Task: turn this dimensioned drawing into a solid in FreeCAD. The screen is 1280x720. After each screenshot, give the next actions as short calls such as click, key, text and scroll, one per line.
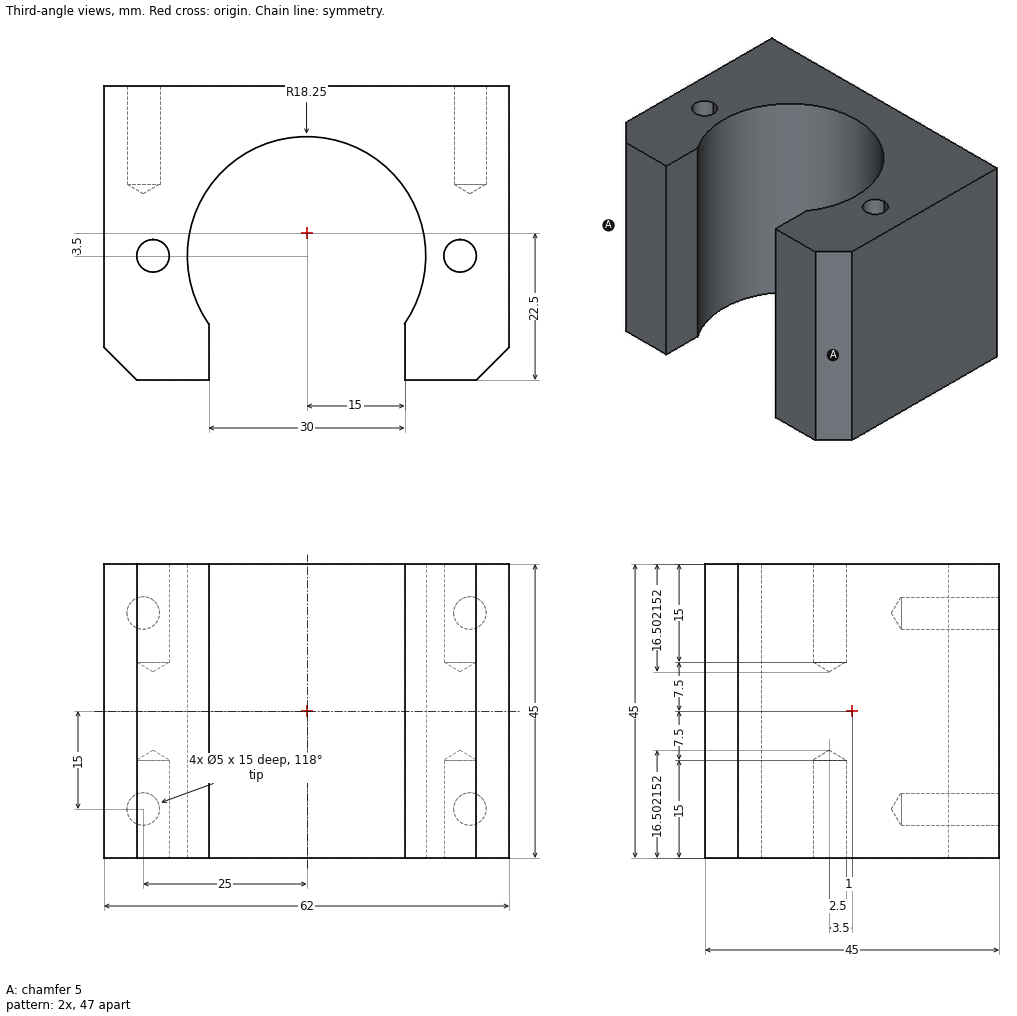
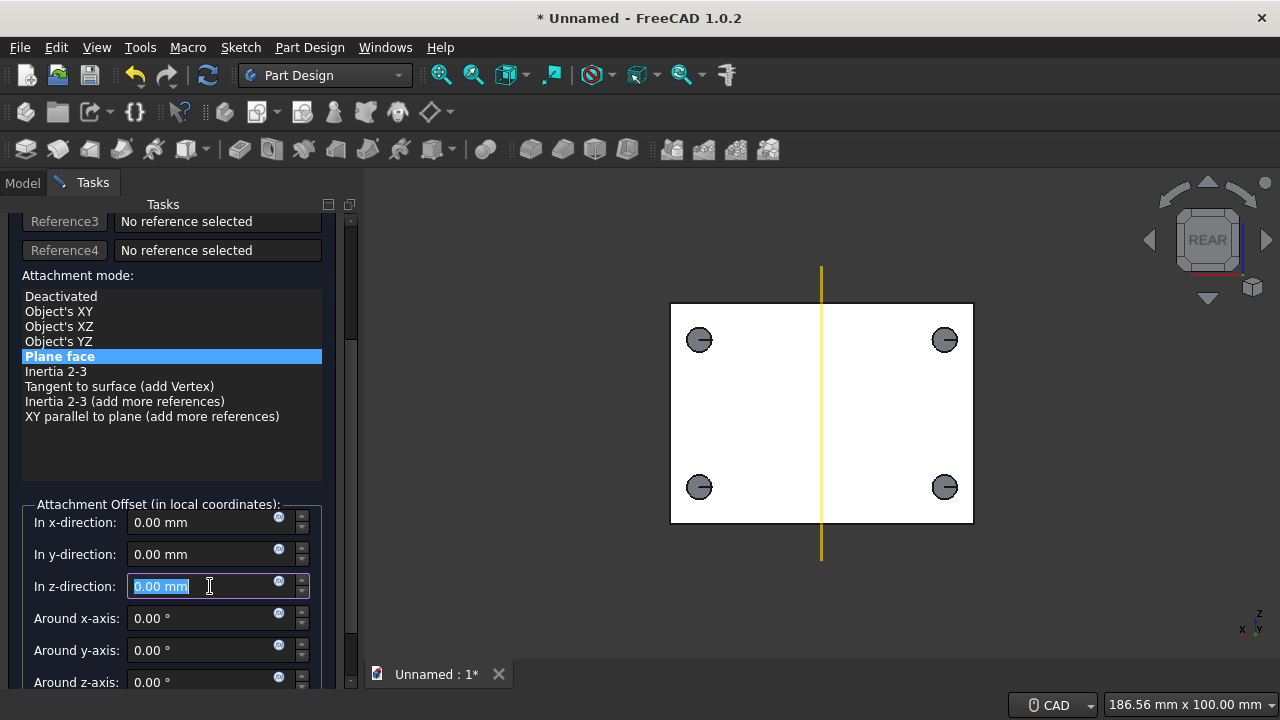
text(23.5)
key(Tab)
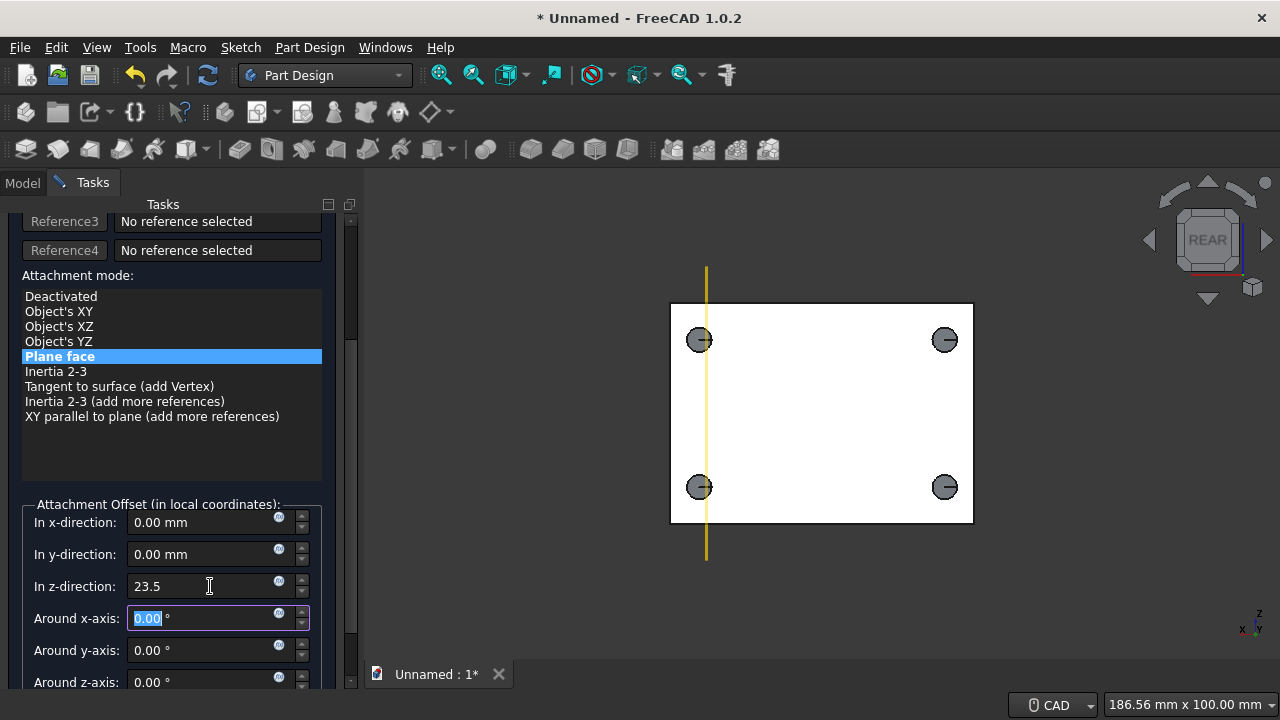
scroll(351, 451, up, 4)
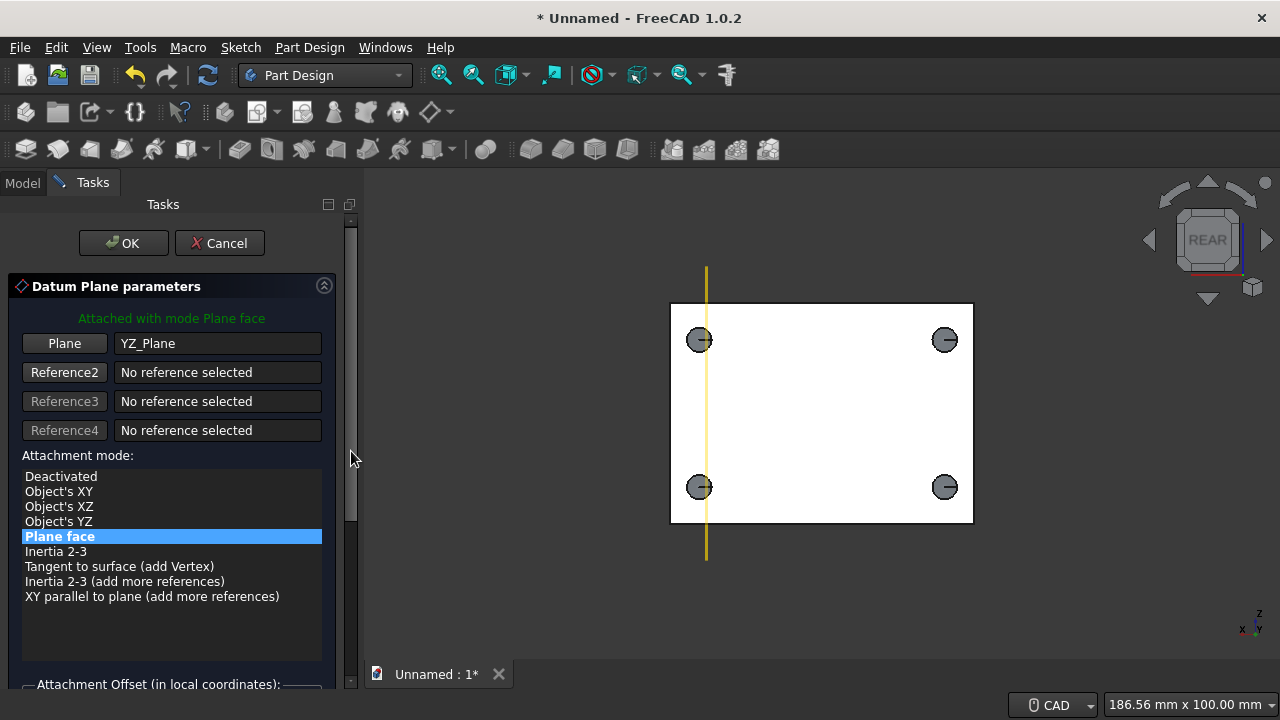
click(124, 243)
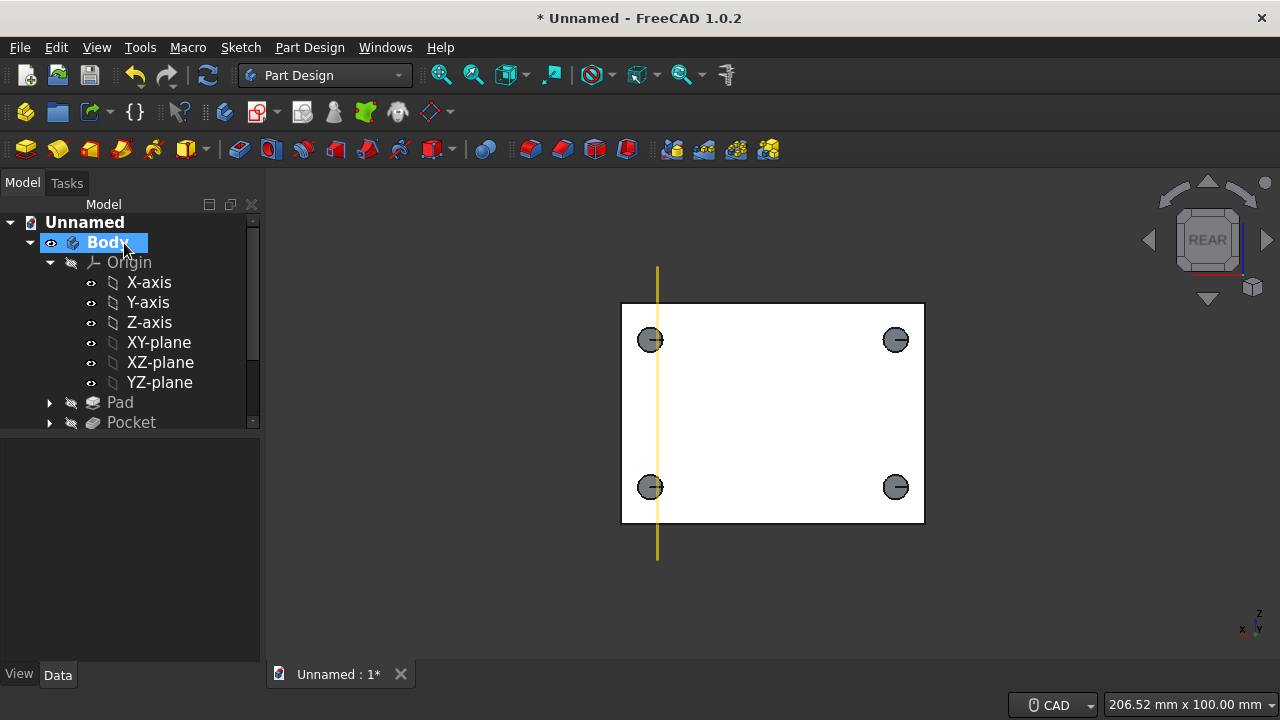
scroll(100, 318, down, 3)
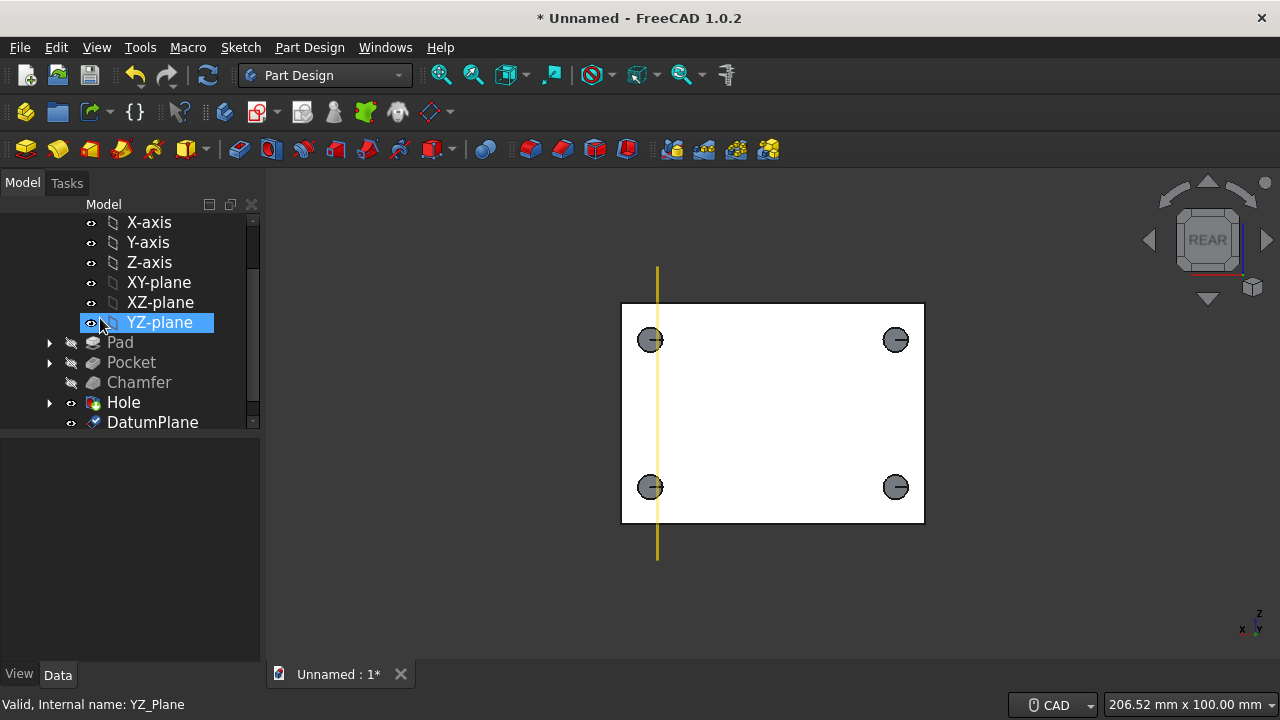
click(116, 403)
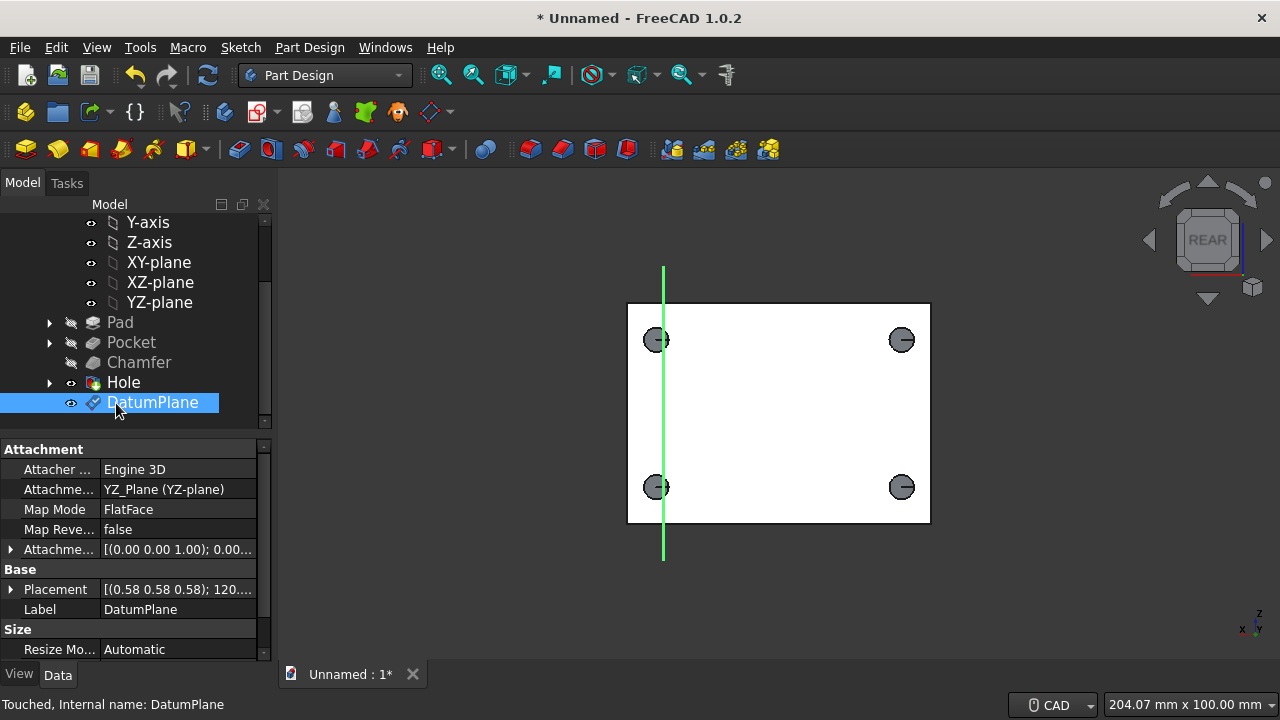
click(258, 112)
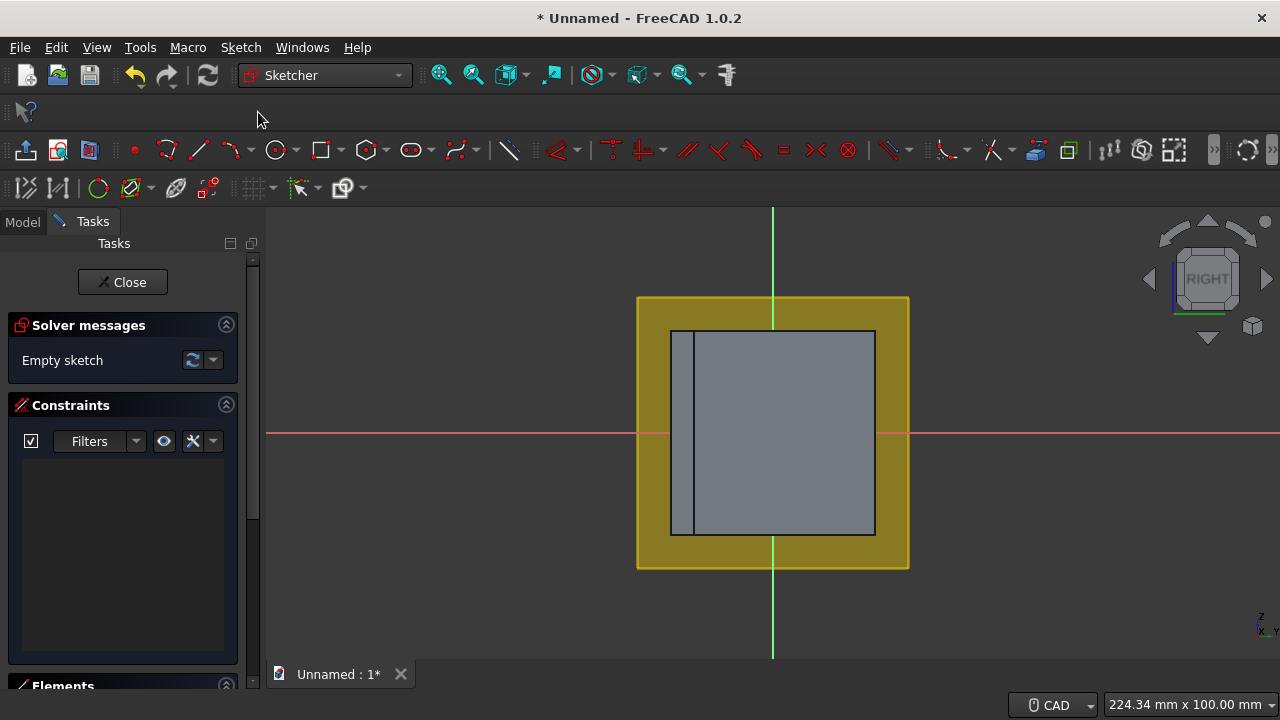
click(90, 150)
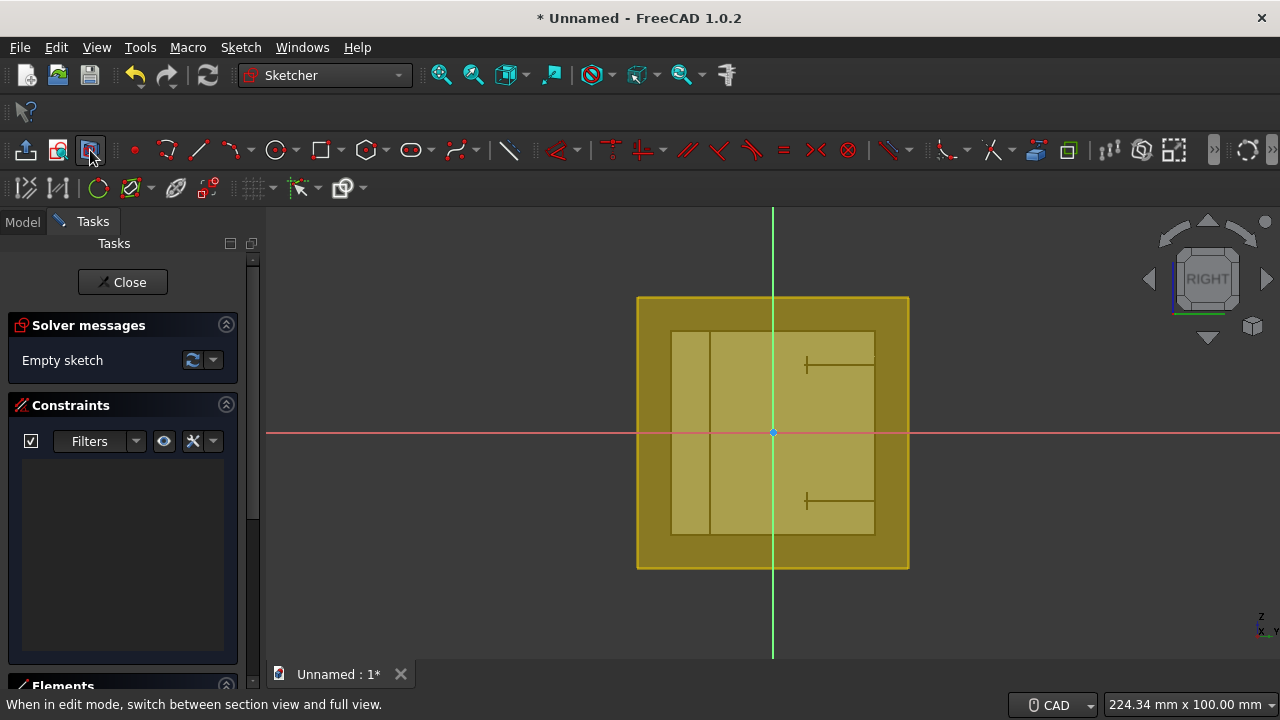
scroll(800, 511, up, 5)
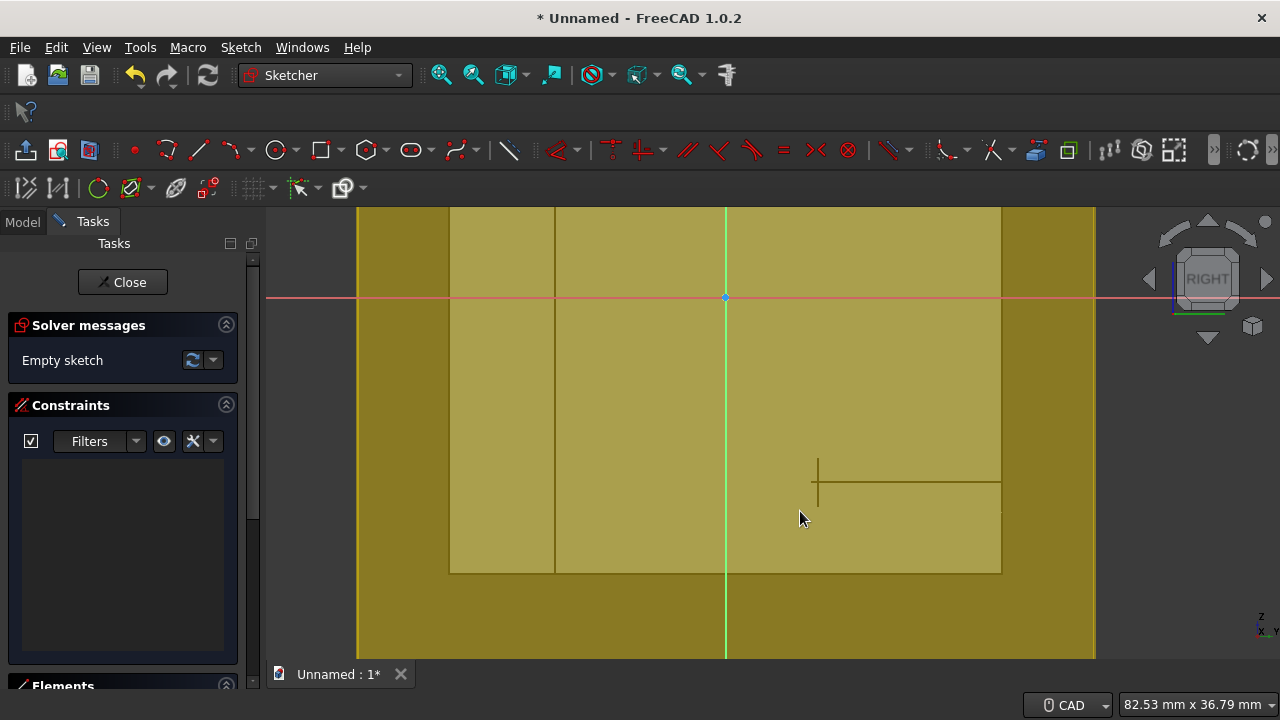
click(168, 150)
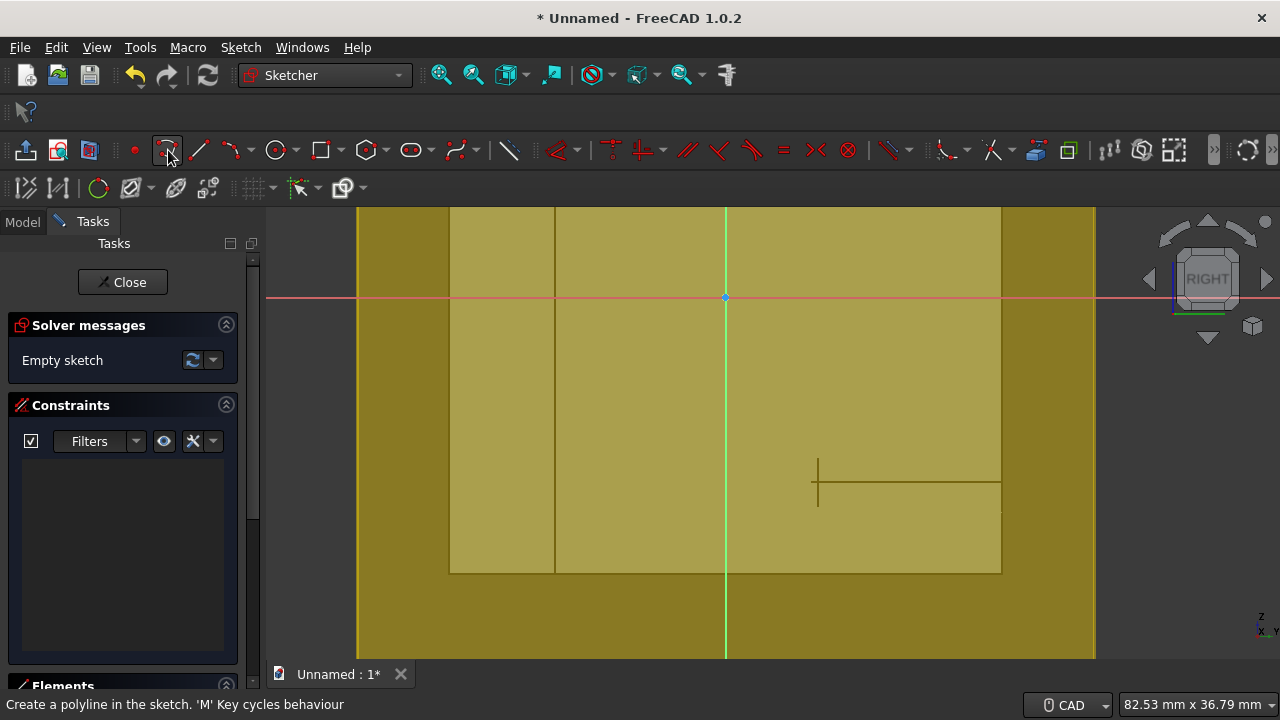
click(683, 372)
click(683, 574)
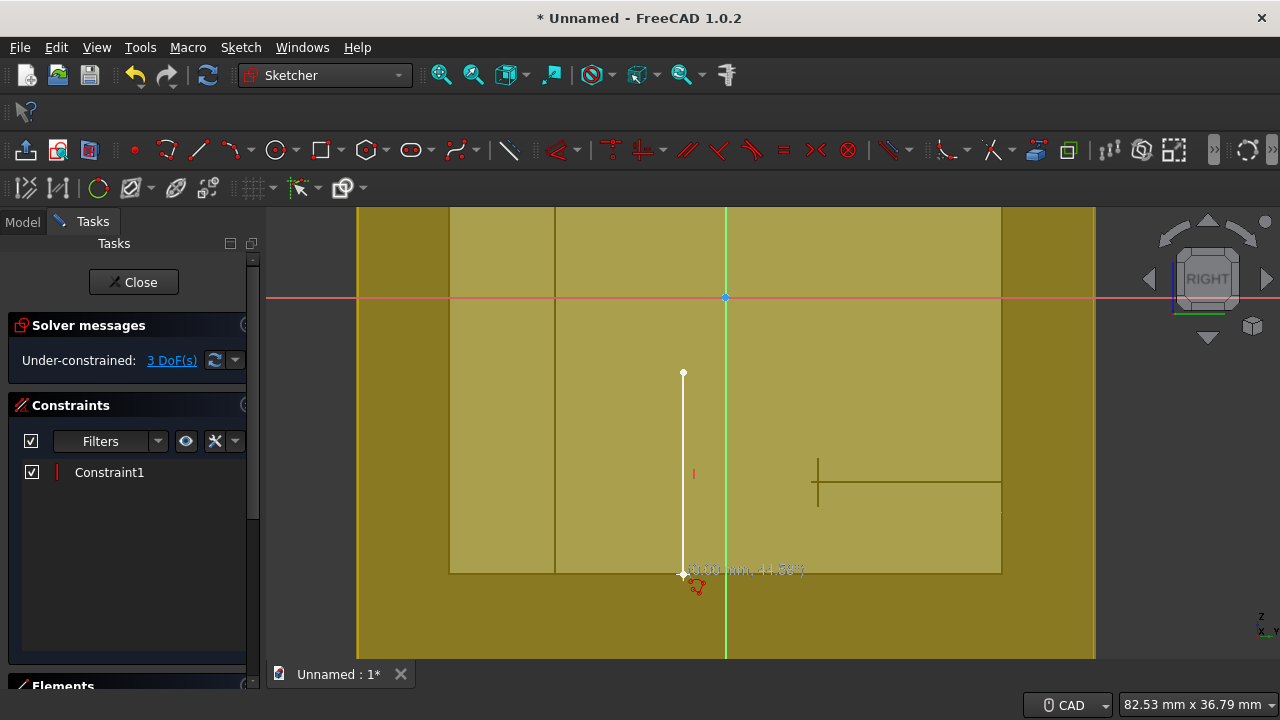
scroll(713, 574, up, 2)